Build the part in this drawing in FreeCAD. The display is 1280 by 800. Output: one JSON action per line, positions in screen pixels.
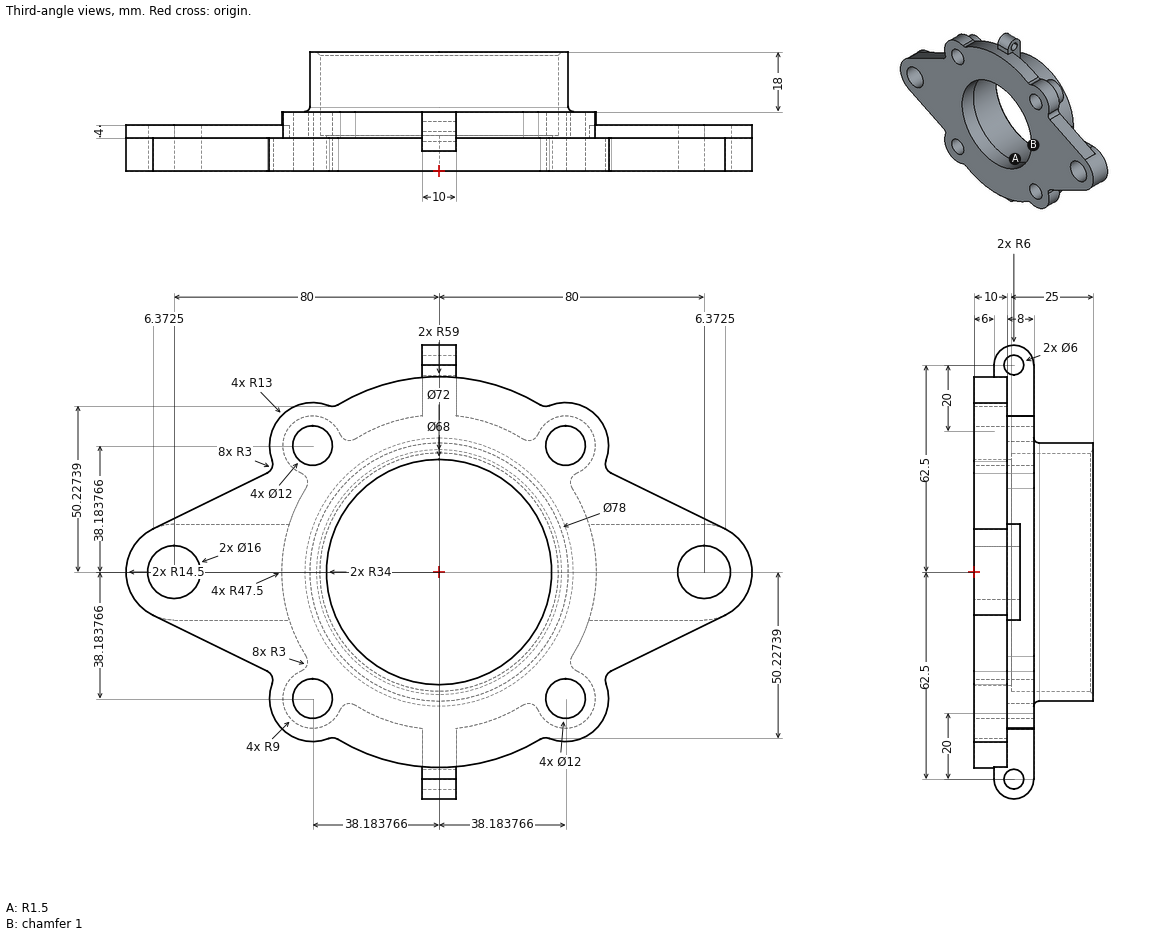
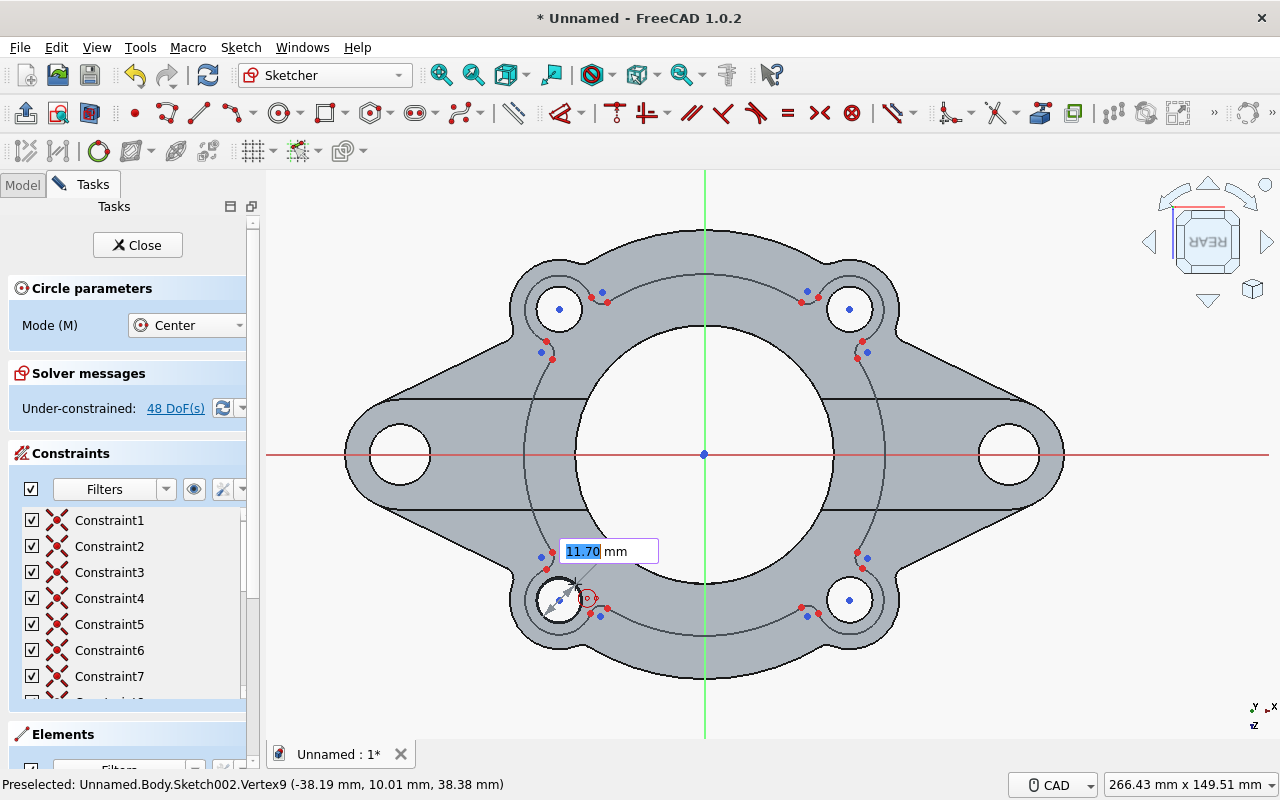
{"action": "type", "text": "12"}
{"action": "key", "text": "Return"}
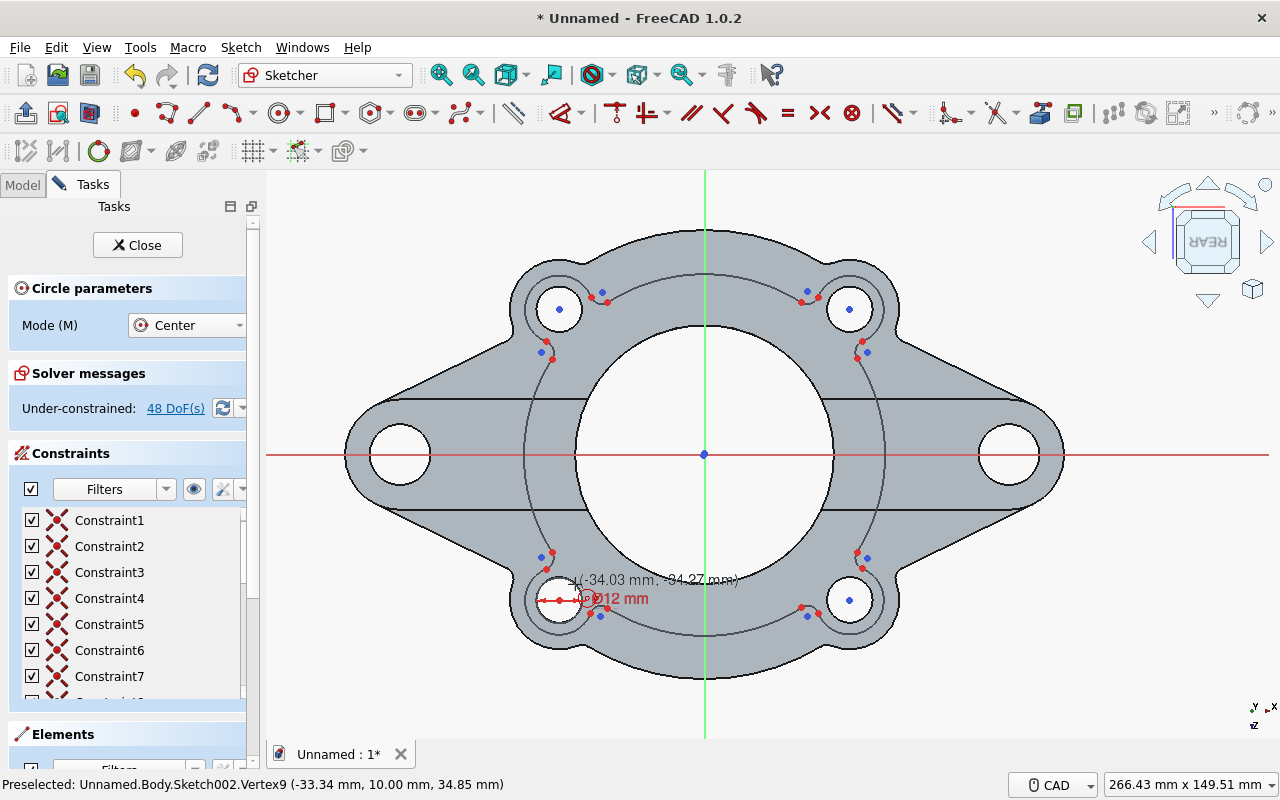
{"action": "left_click", "coordinate": [850, 600]}
{"action": "mouse_move", "coordinate": [834, 584]}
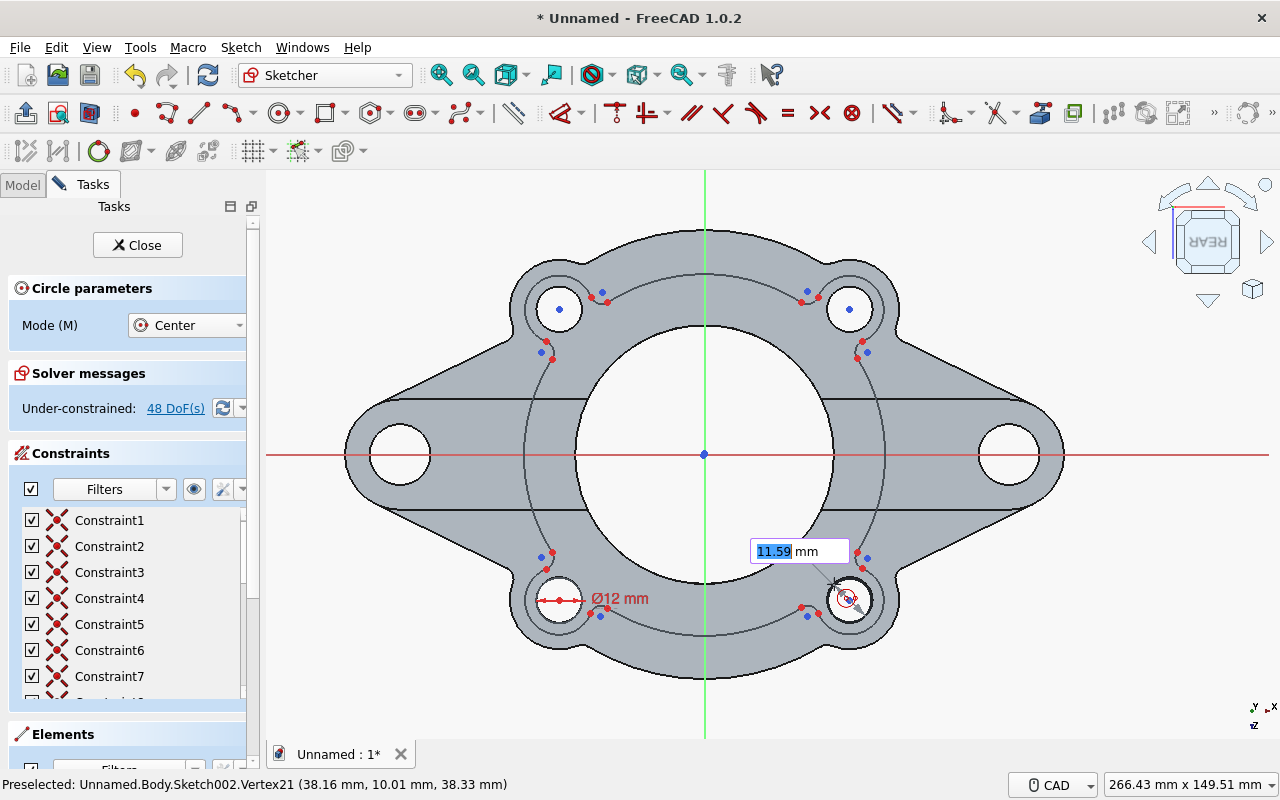
{"action": "type", "text": "12"}
{"action": "key", "text": "Return"}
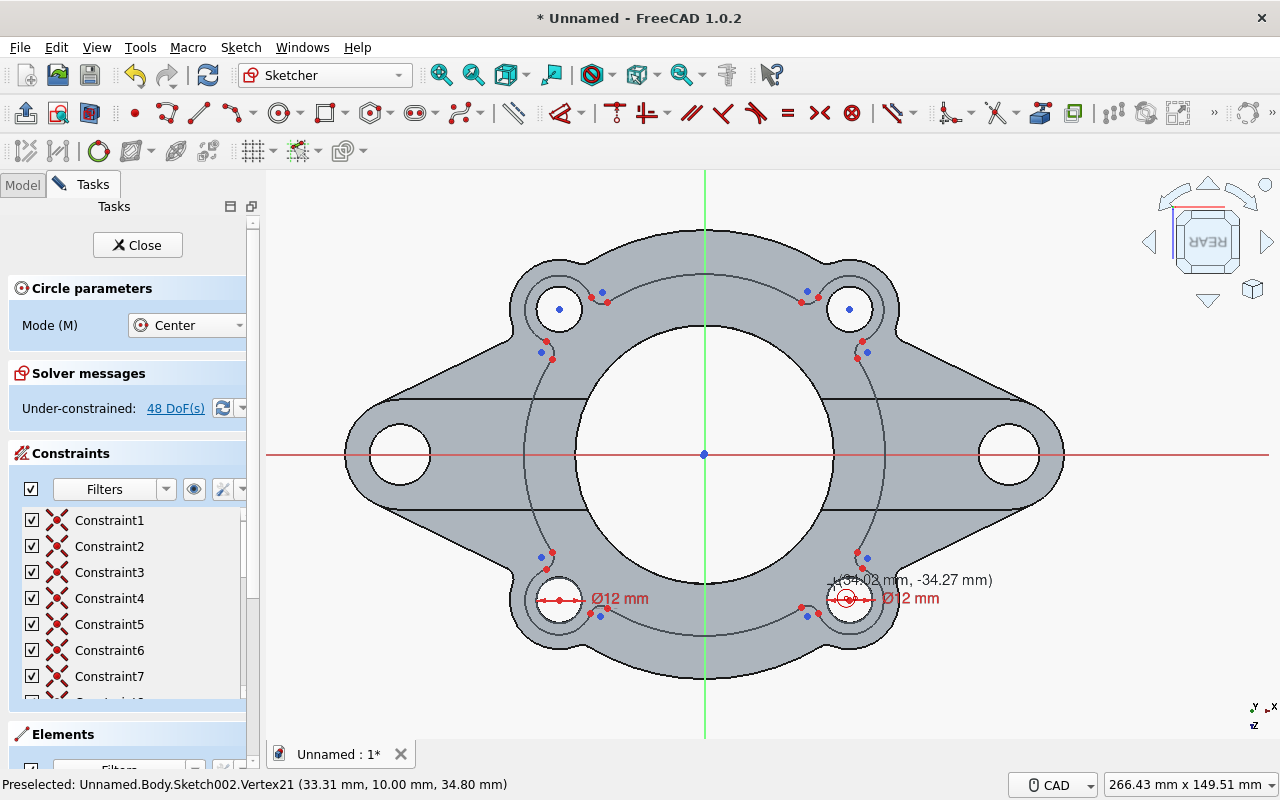
{"action": "left_click", "coordinate": [559, 309]}
{"action": "mouse_move", "coordinate": [575, 325]}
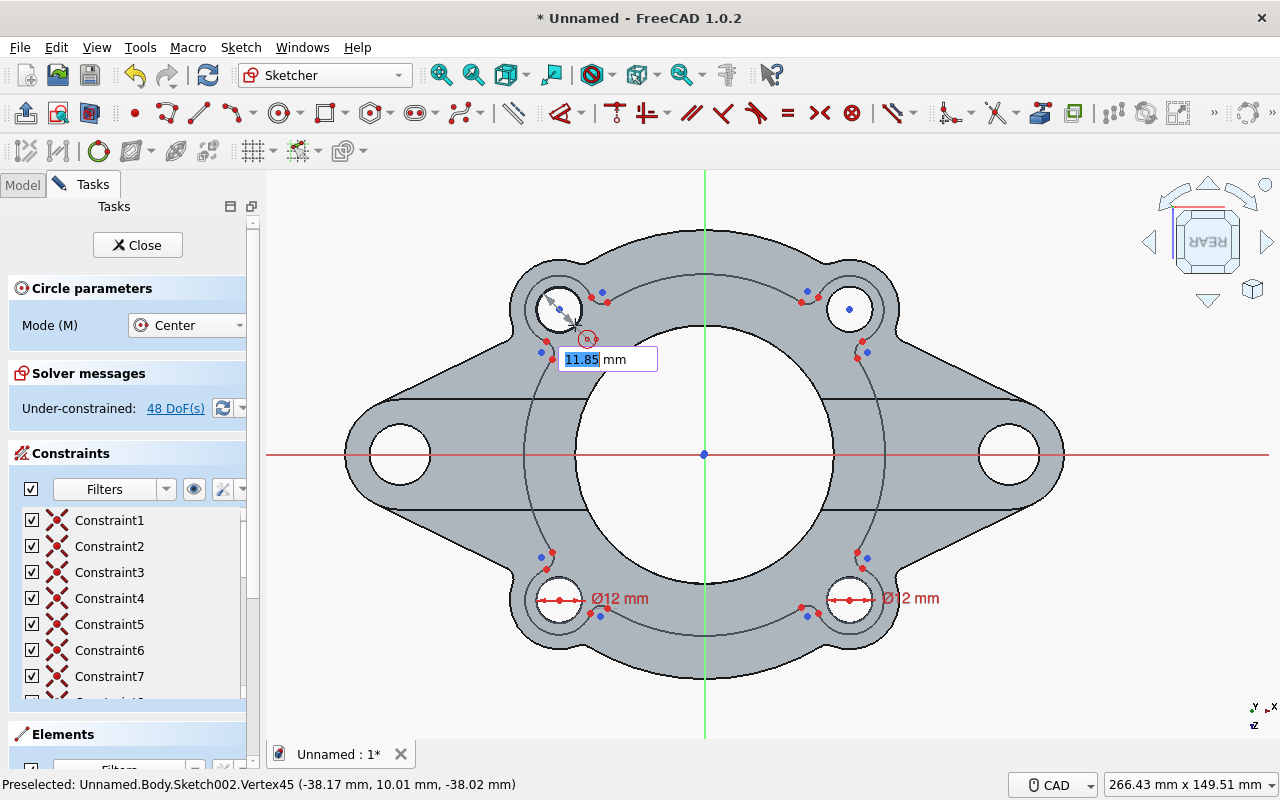
{"action": "type", "text": "12"}
{"action": "key", "text": "Return"}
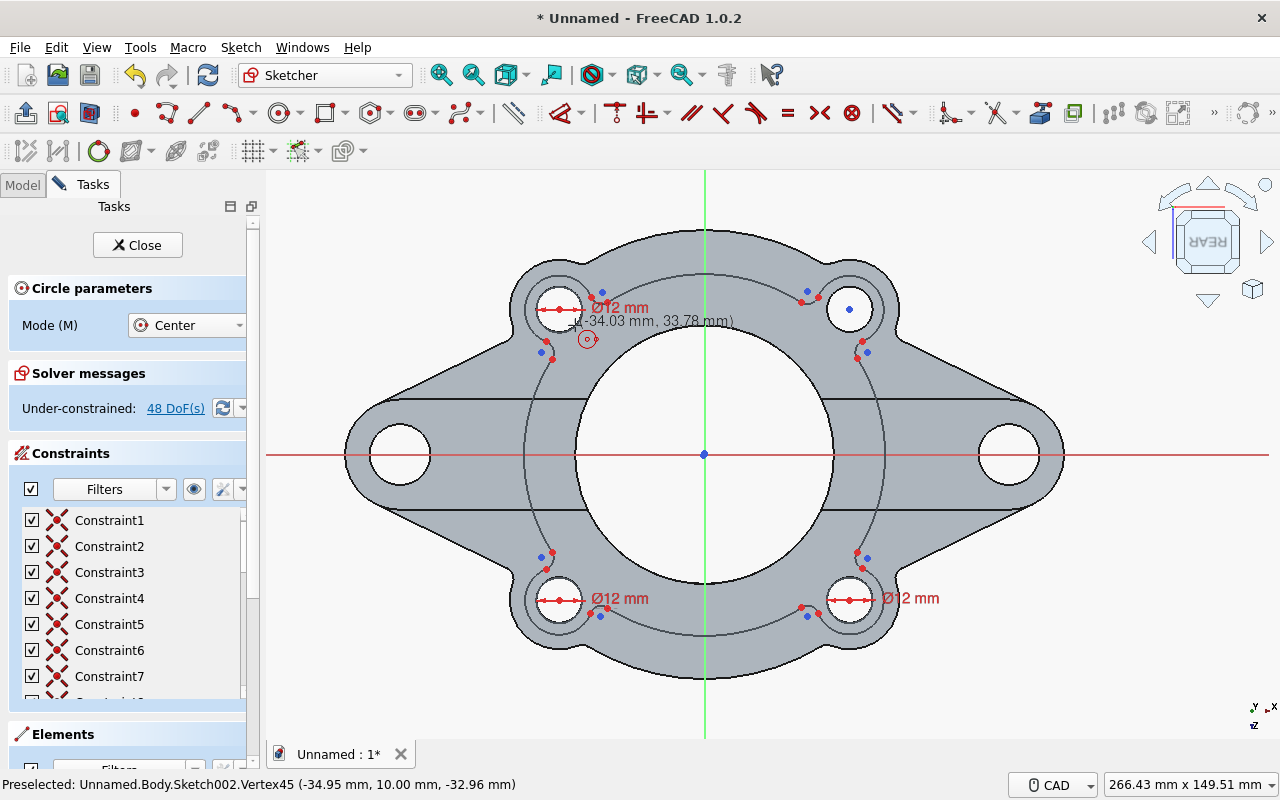
{"action": "left_click", "coordinate": [705, 455]}
{"action": "mouse_move", "coordinate": [796, 363]}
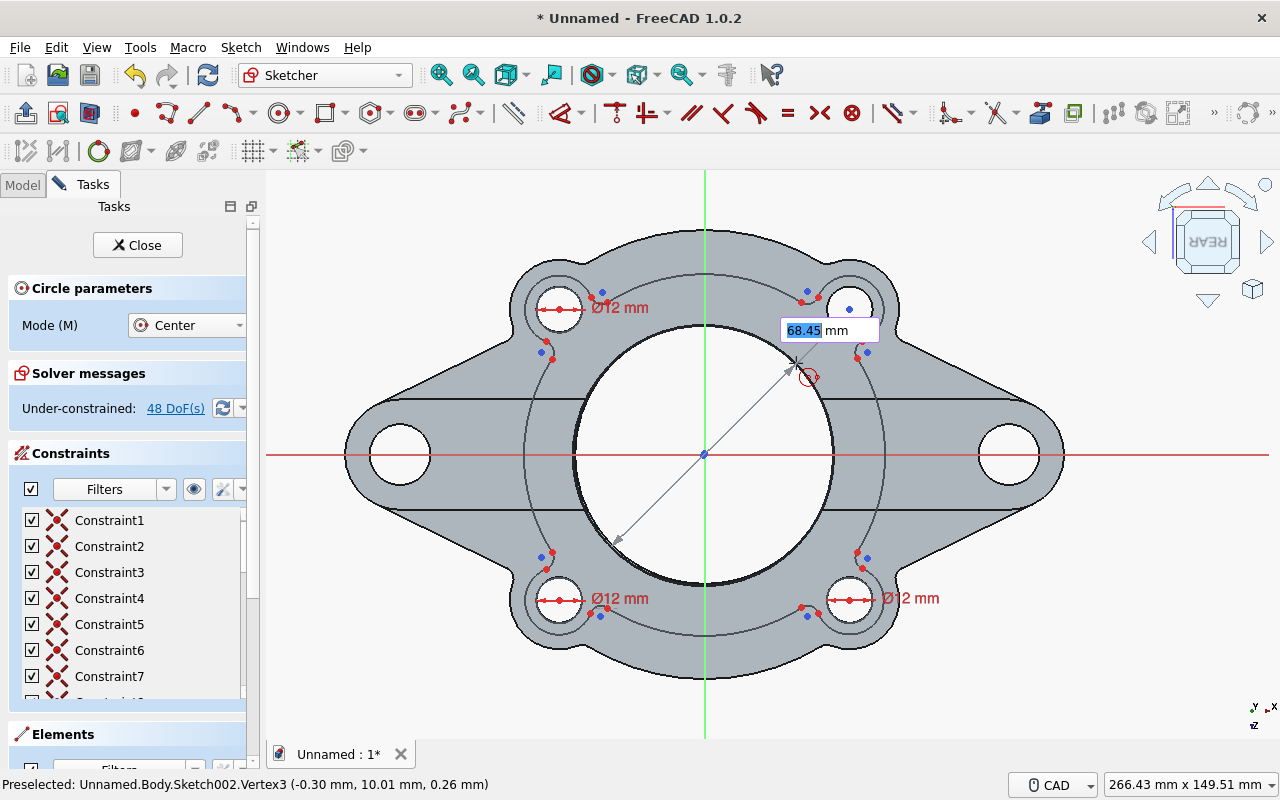
{"action": "type", "text": "68"}
{"action": "key", "text": "Return"}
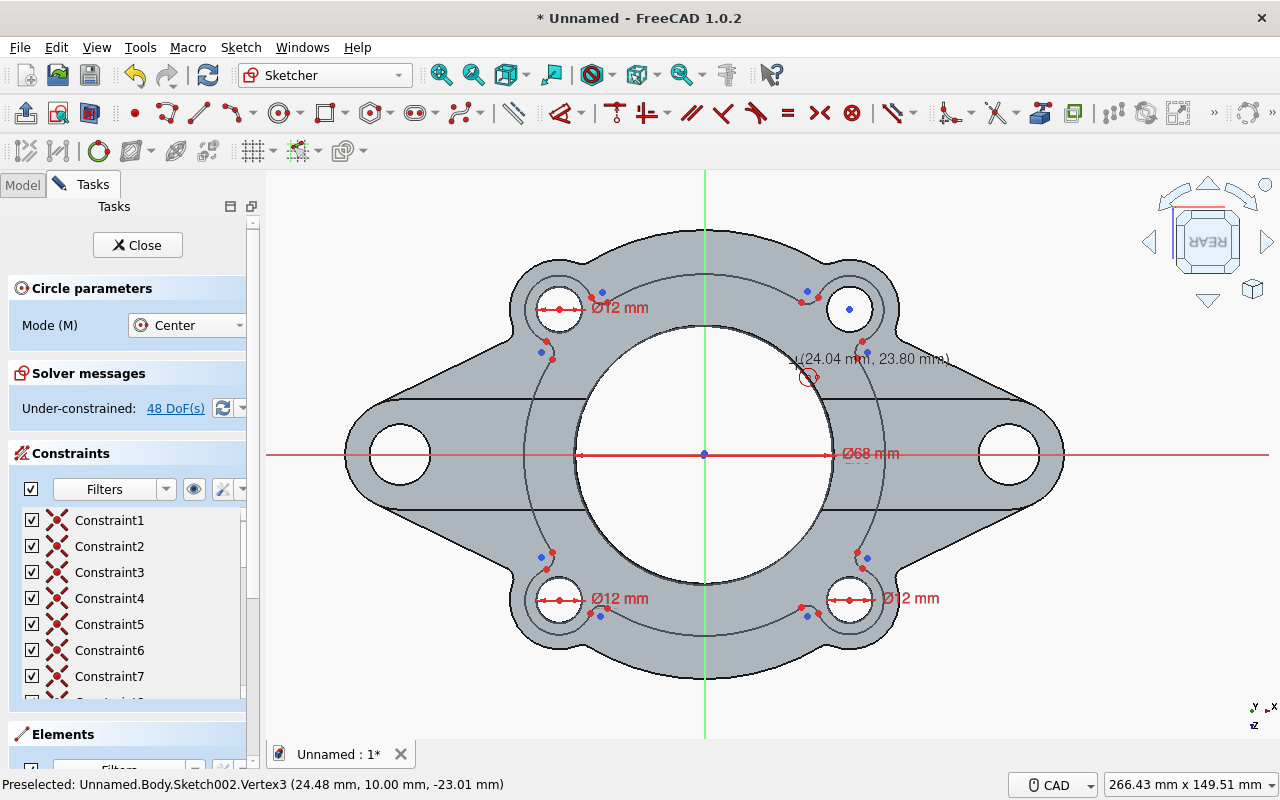
{"action": "left_click", "coordinate": [850, 309]}
{"action": "mouse_move", "coordinate": [834, 325]}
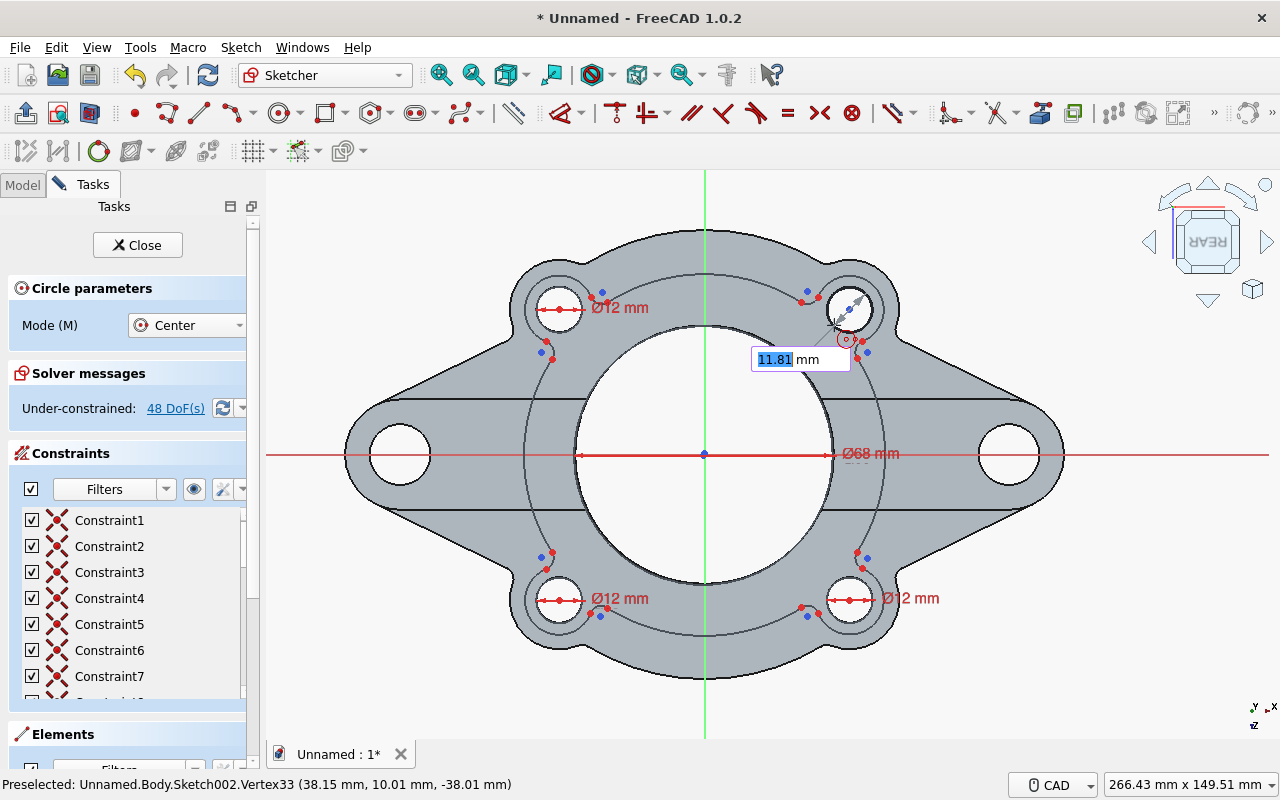
{"action": "type", "text": "12"}
{"action": "key", "text": "Return"}
{"action": "key", "text": "Escape"}